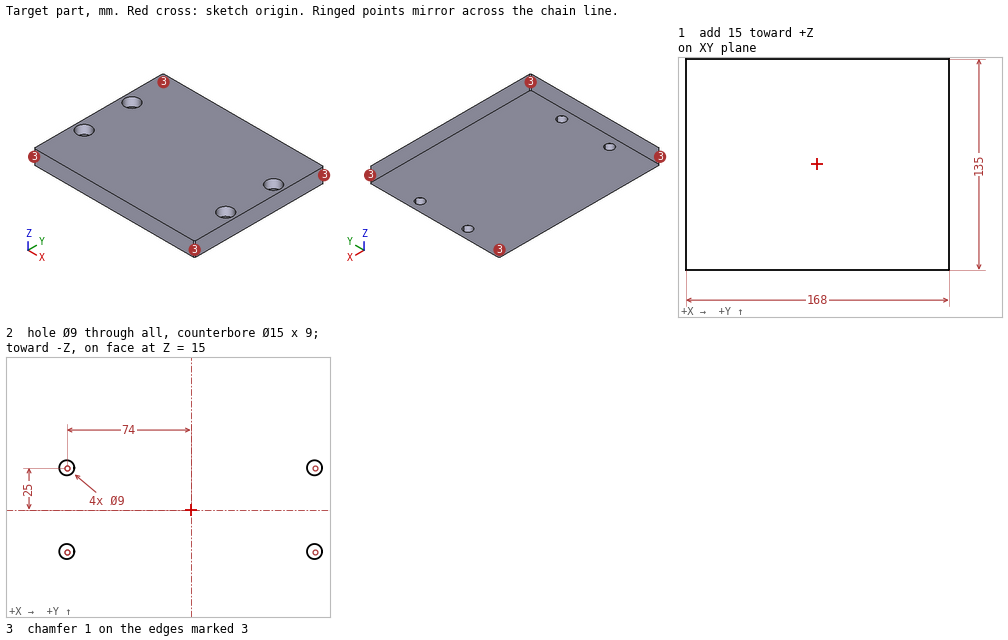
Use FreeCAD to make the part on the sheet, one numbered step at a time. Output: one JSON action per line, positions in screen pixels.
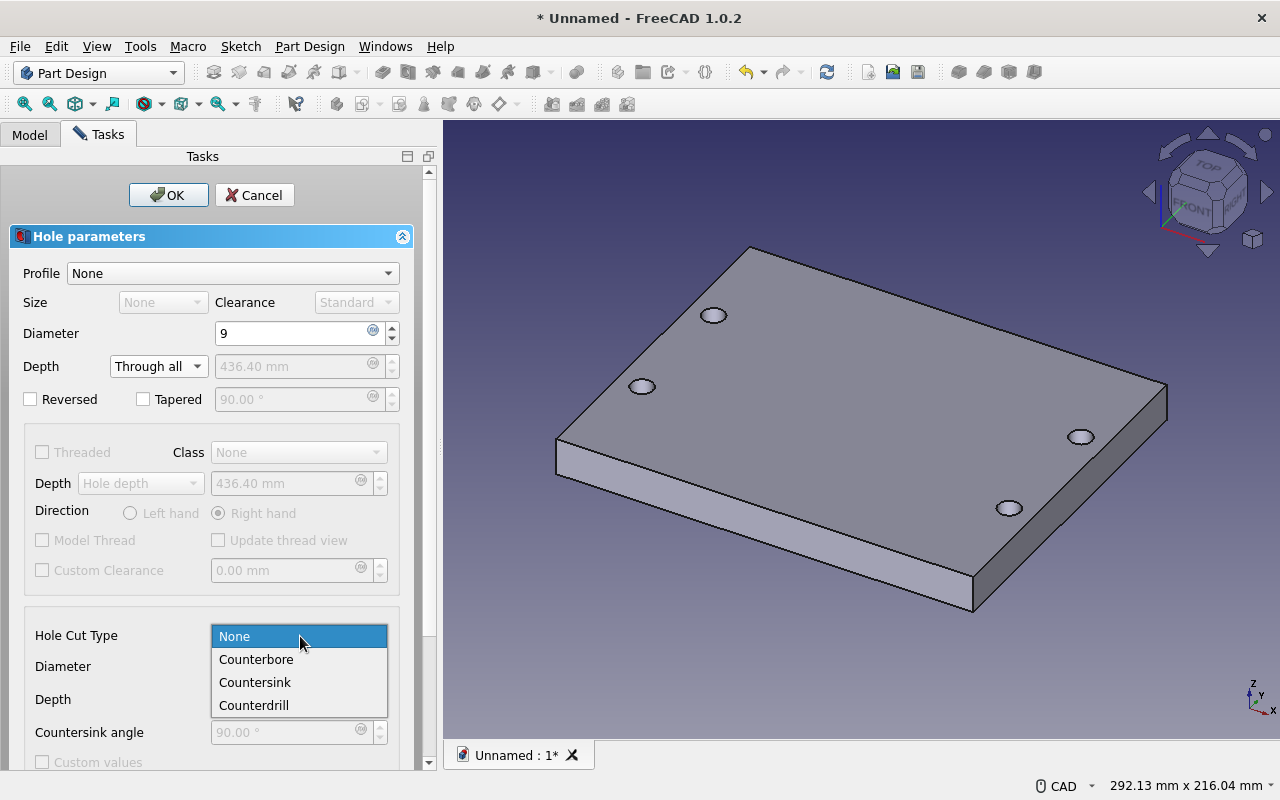
{"action": "left_click", "coordinate": [298, 660]}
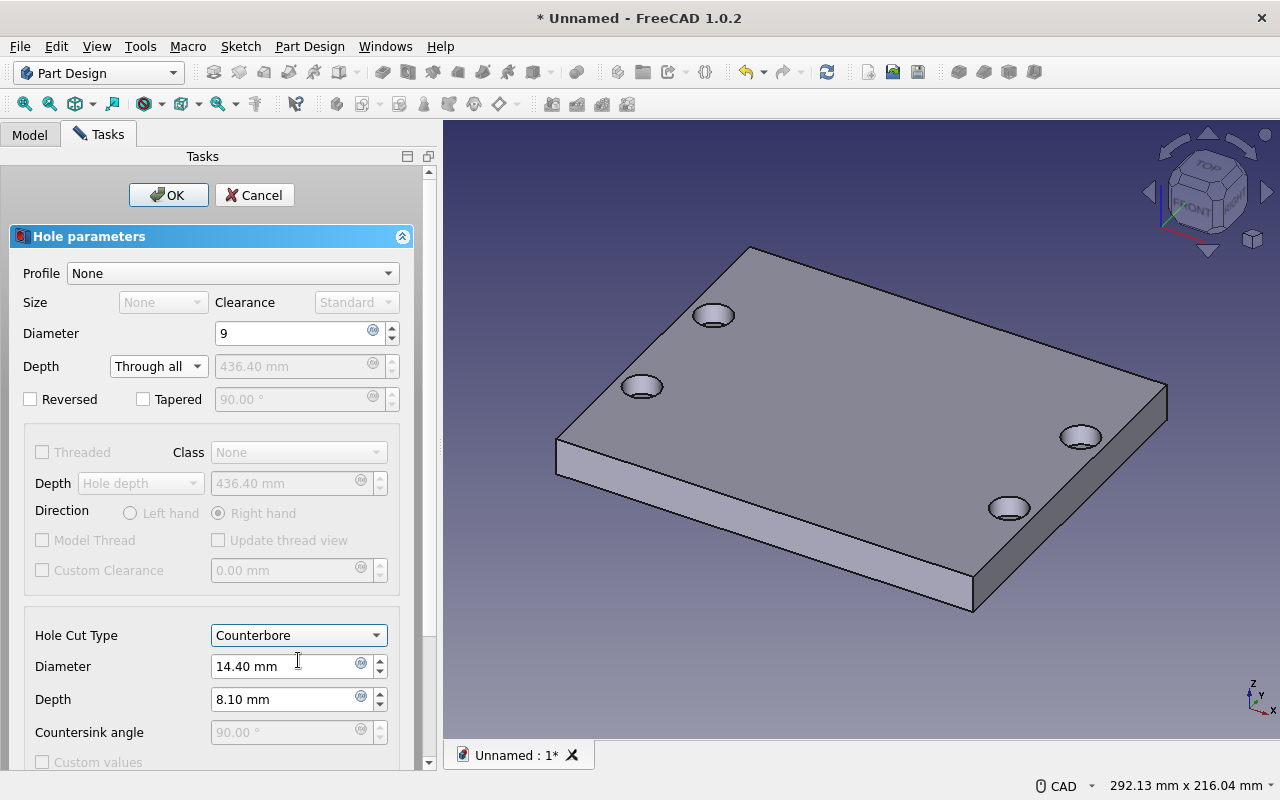
{"action": "triple_click", "coordinate": [292, 666]}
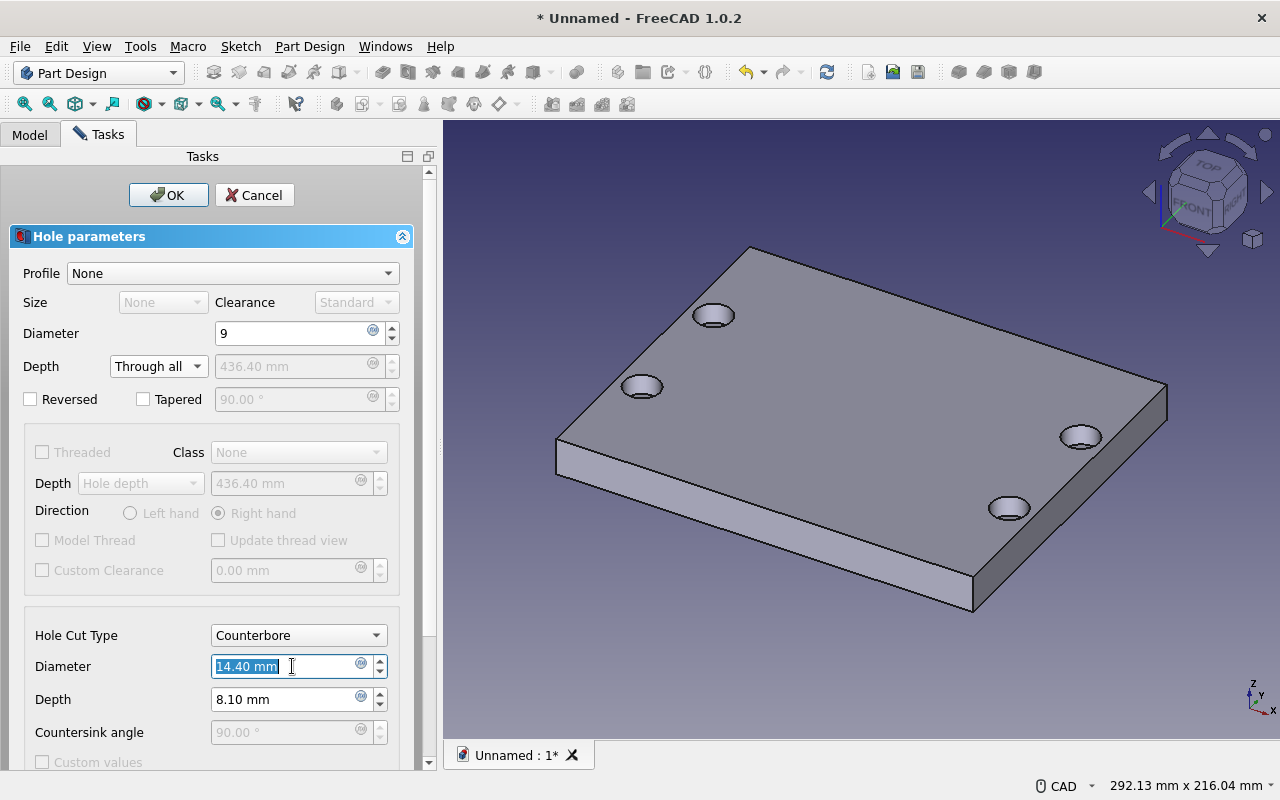
{"action": "type", "text": "15"}
{"action": "key", "text": "Tab"}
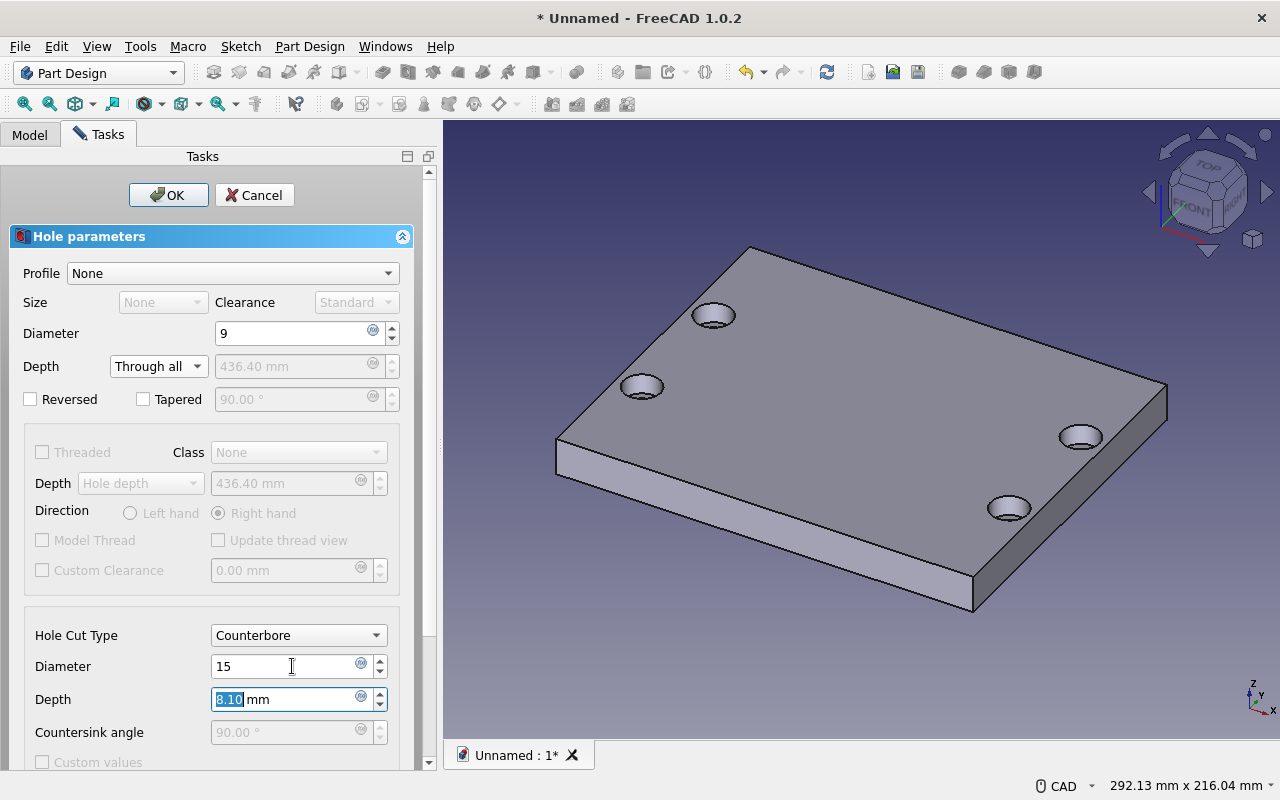
{"action": "type", "text": "9"}
{"action": "key", "text": "Tab"}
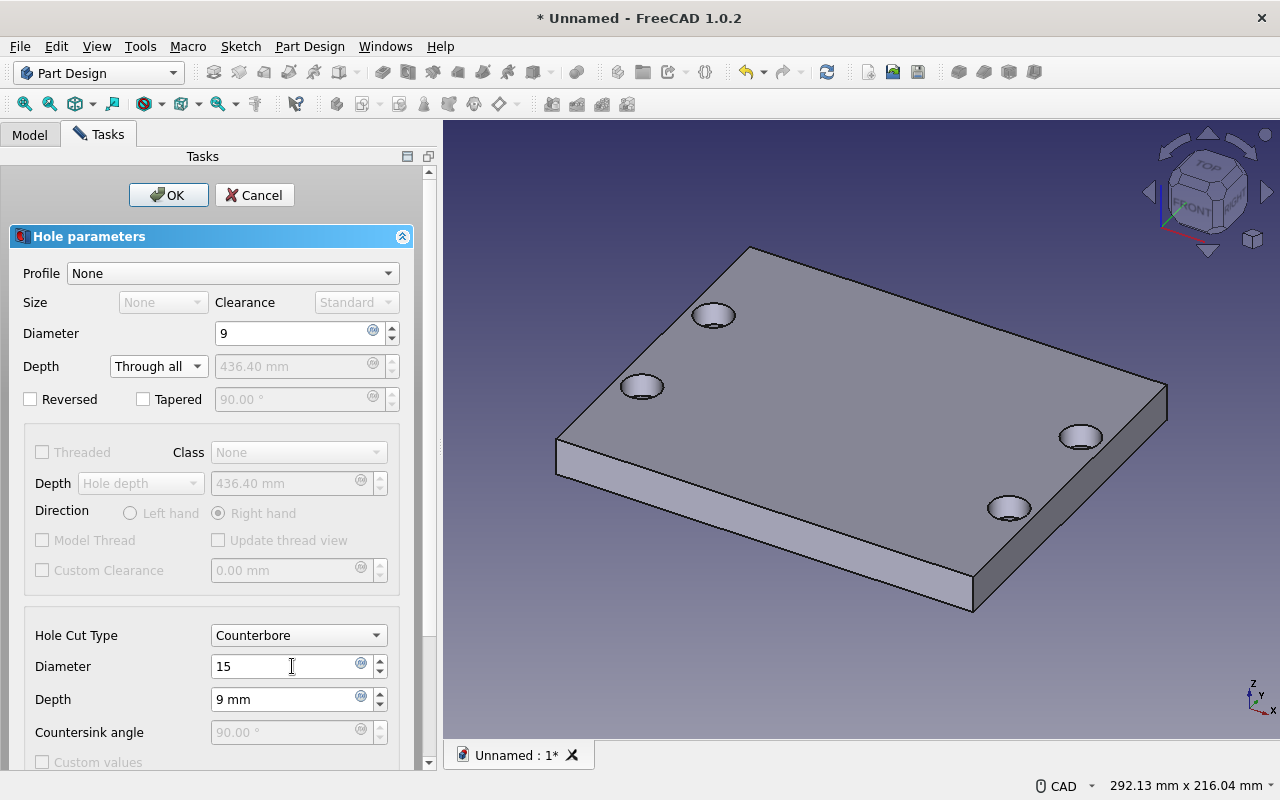
{"action": "left_click", "coordinate": [169, 195]}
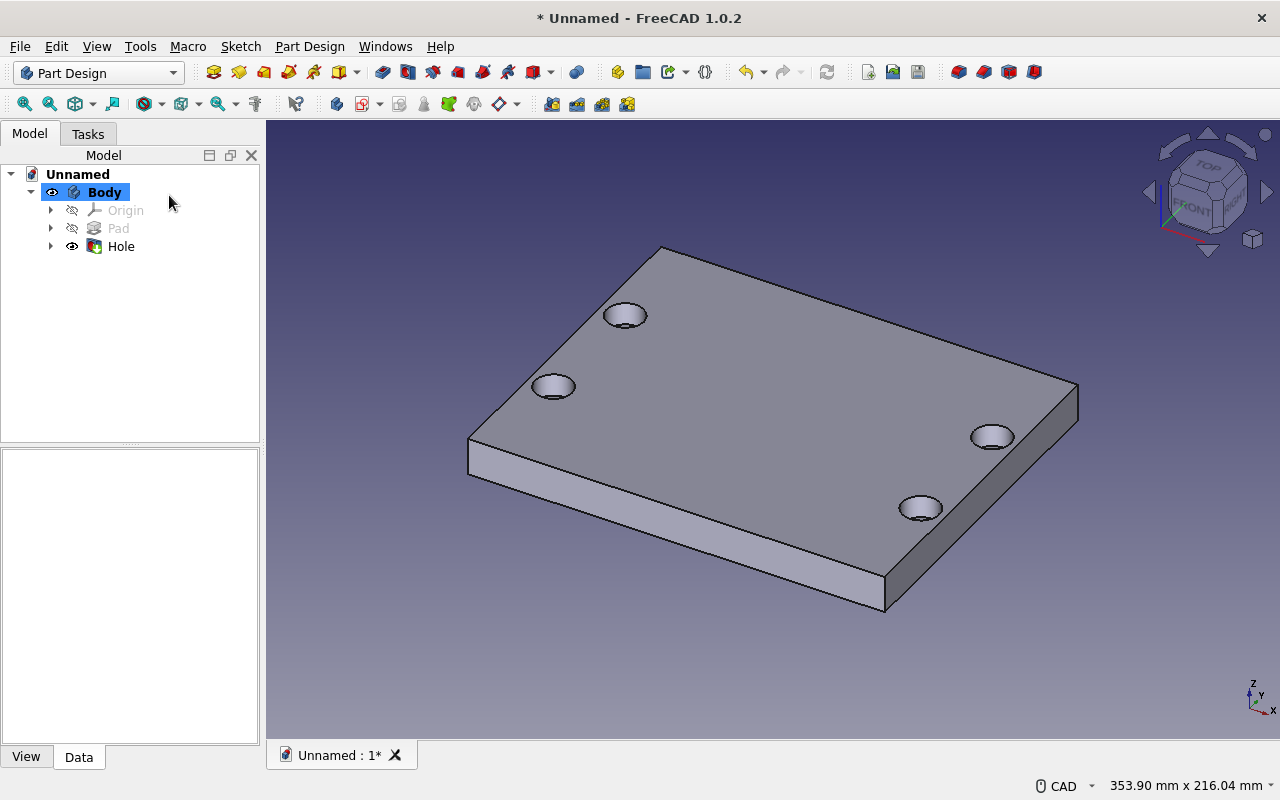
{"action": "left_click", "coordinate": [885, 594]}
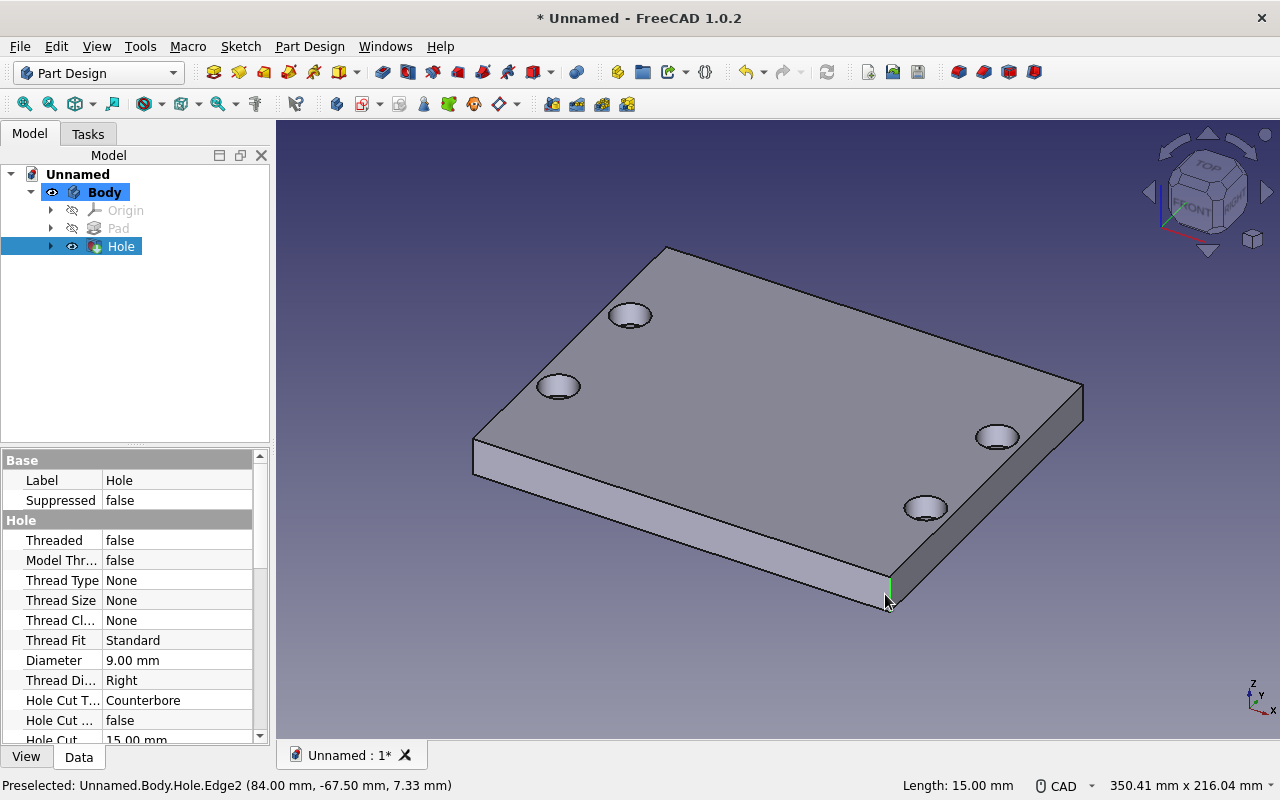
{"action": "key", "text": "0"}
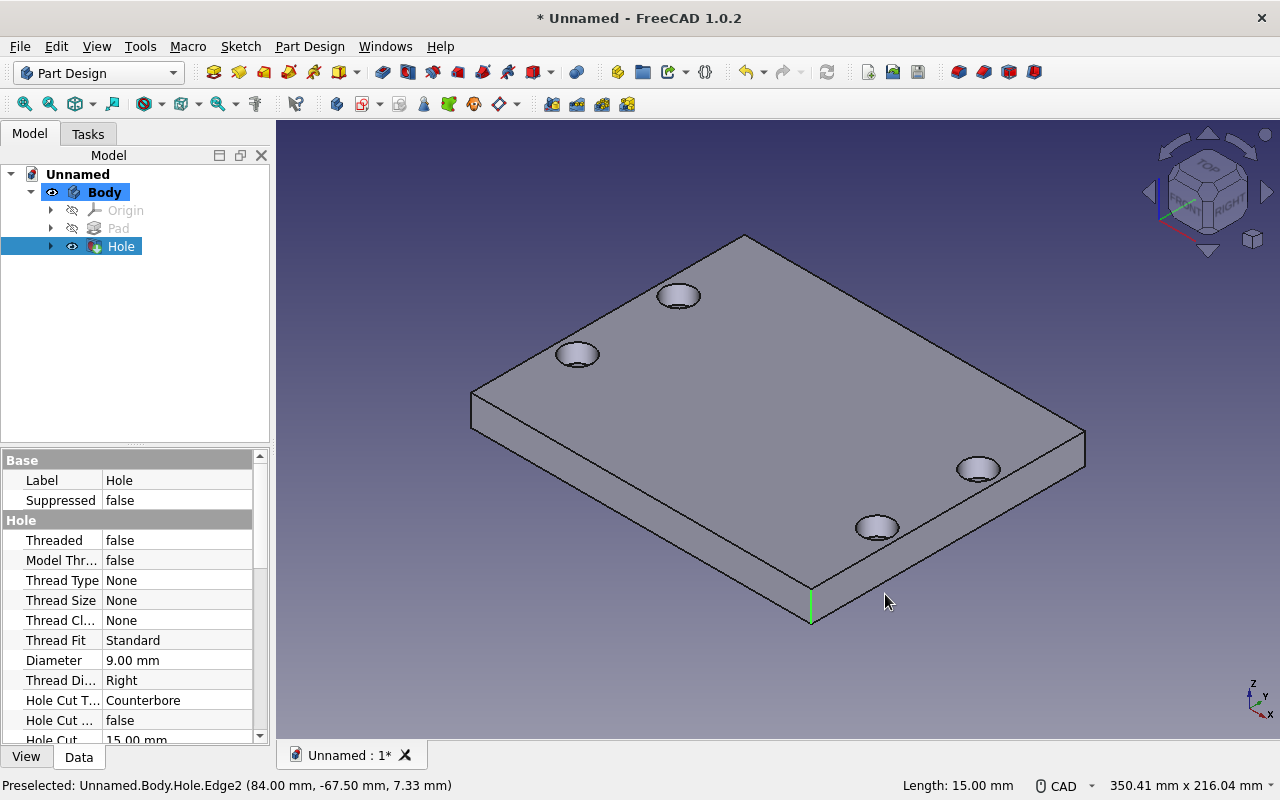
{"action": "key", "text": "2"}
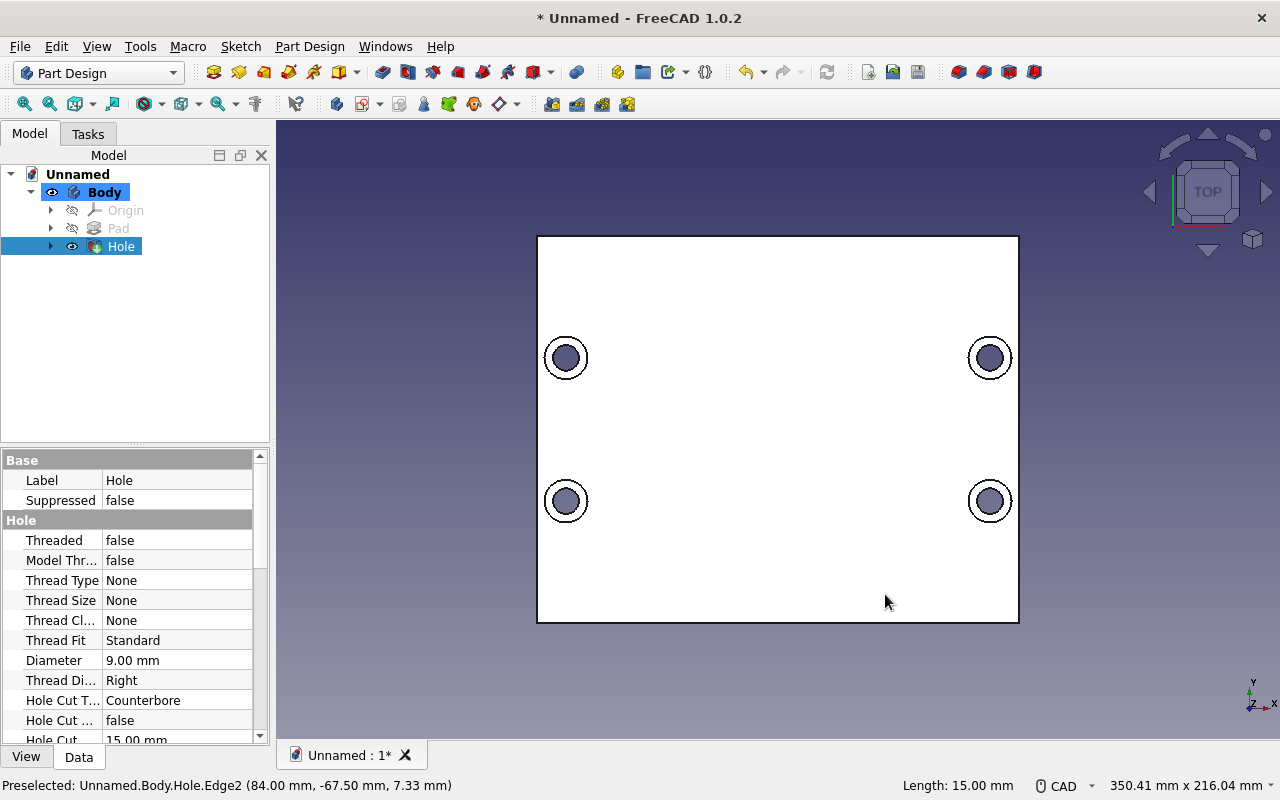
{"action": "key", "text": "1"}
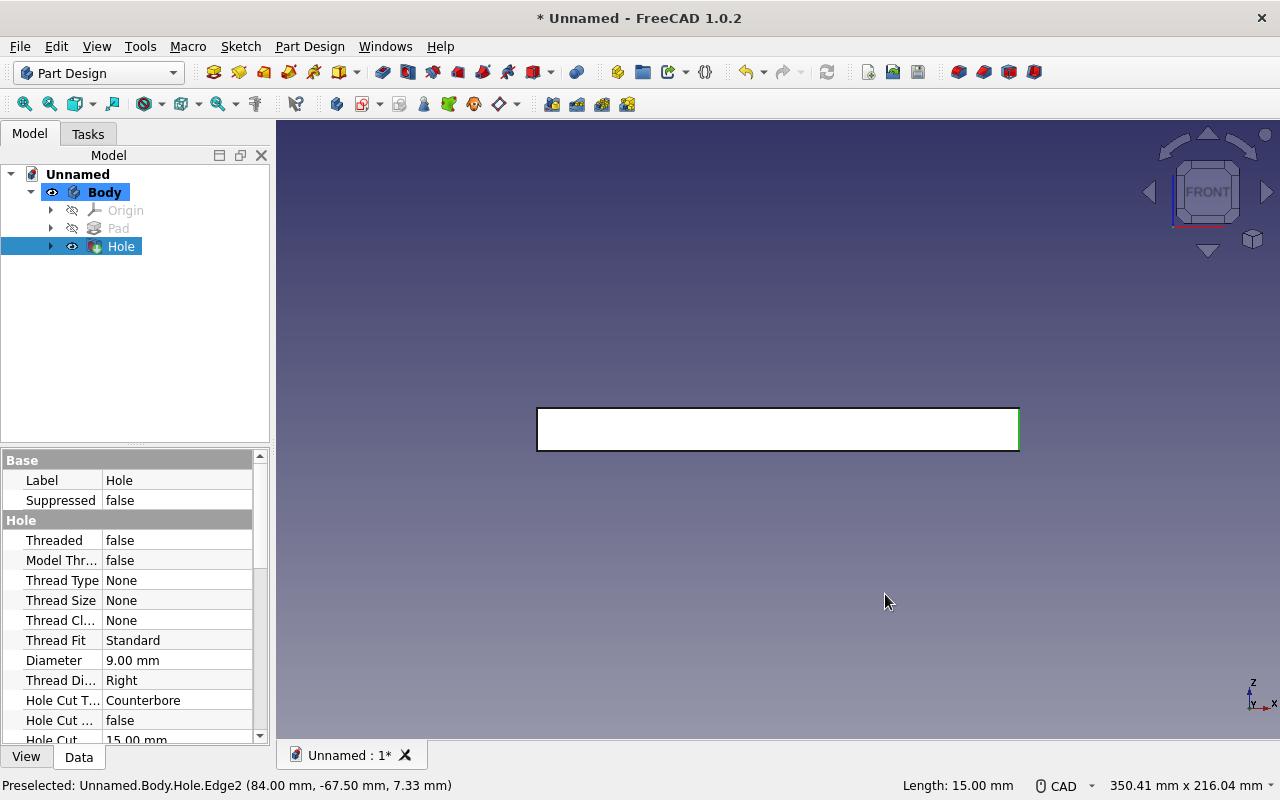
{"action": "left_click", "coordinate": [537, 429], "text": "ctrl"}